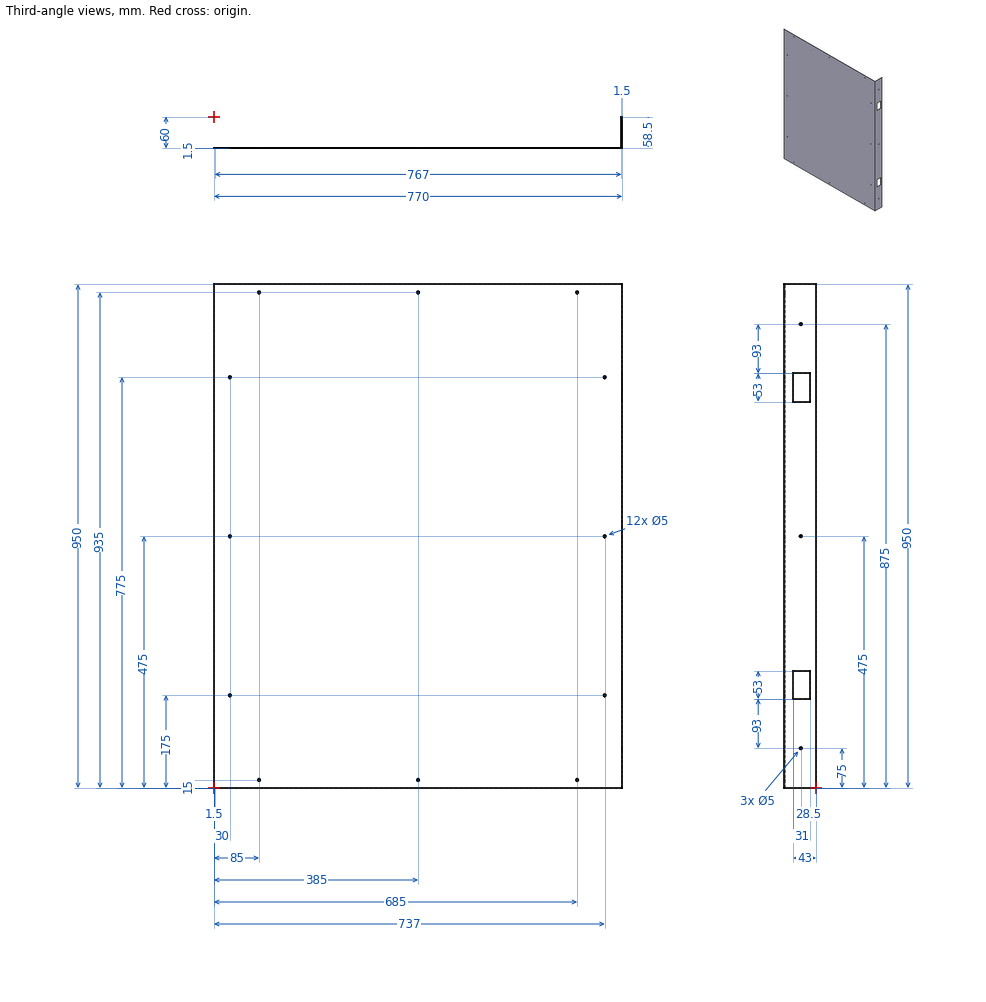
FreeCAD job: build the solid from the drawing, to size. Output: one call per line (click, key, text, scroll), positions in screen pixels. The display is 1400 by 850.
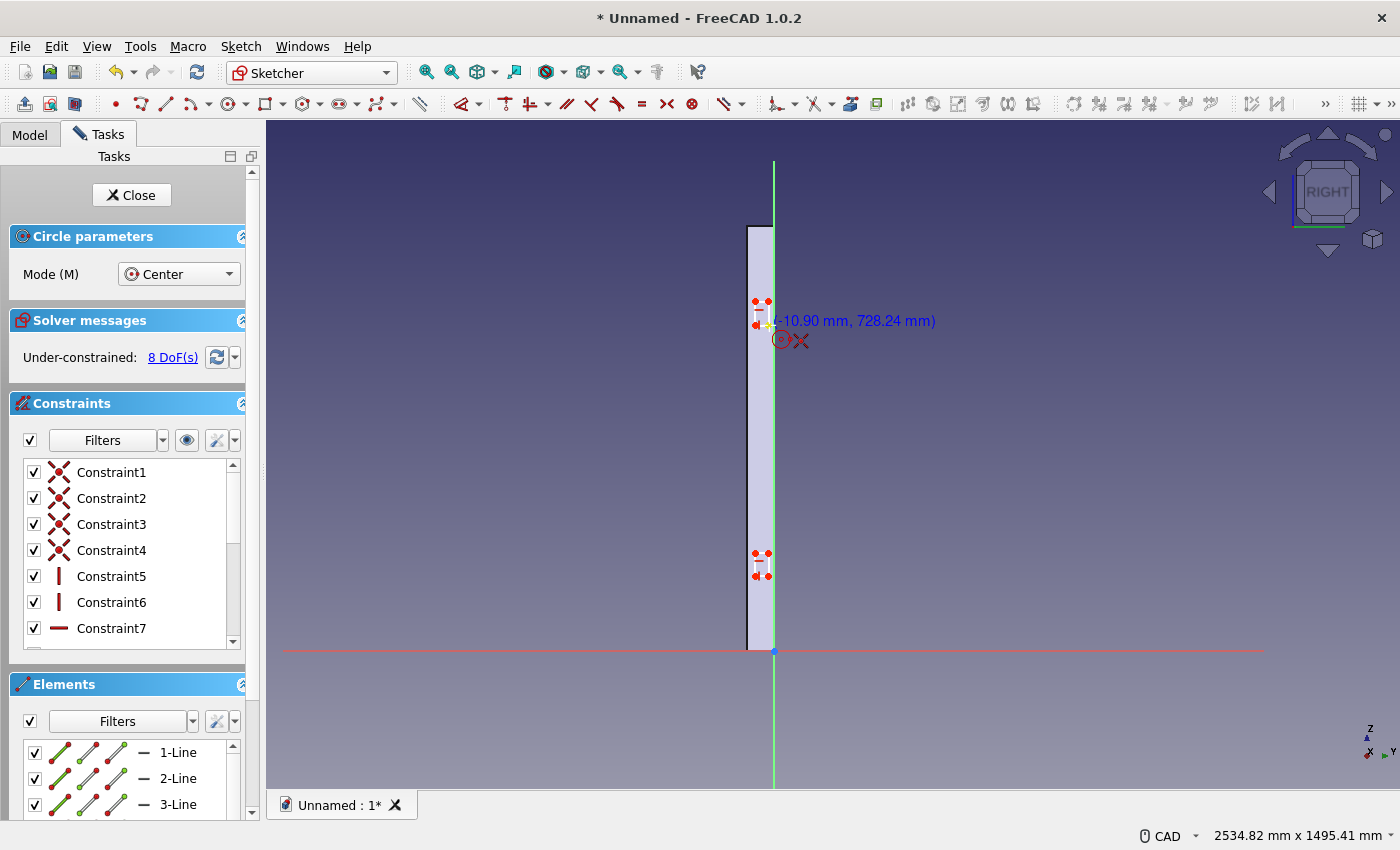
scroll(761, 618, up, 16)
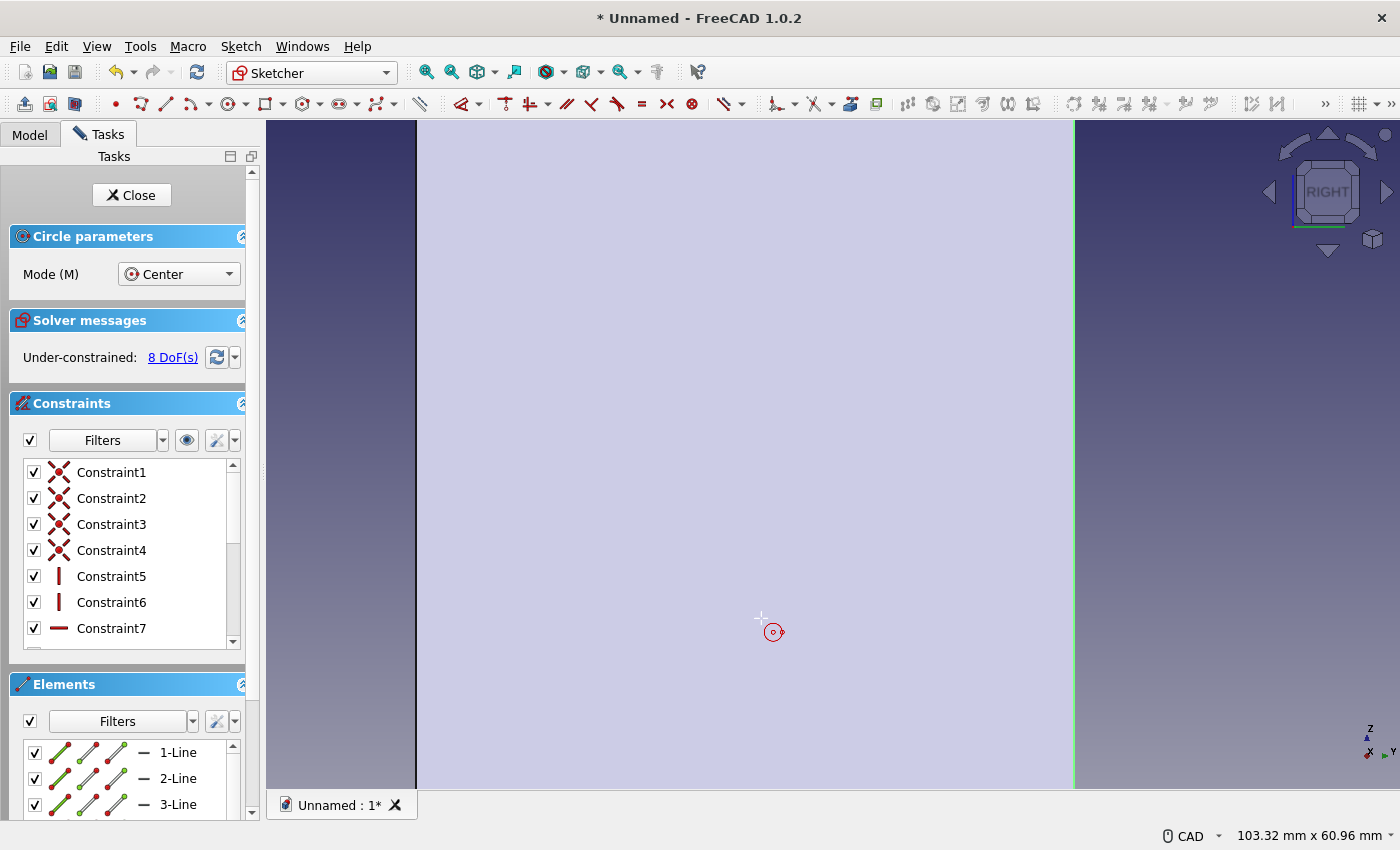
scroll(761, 656, down, 15)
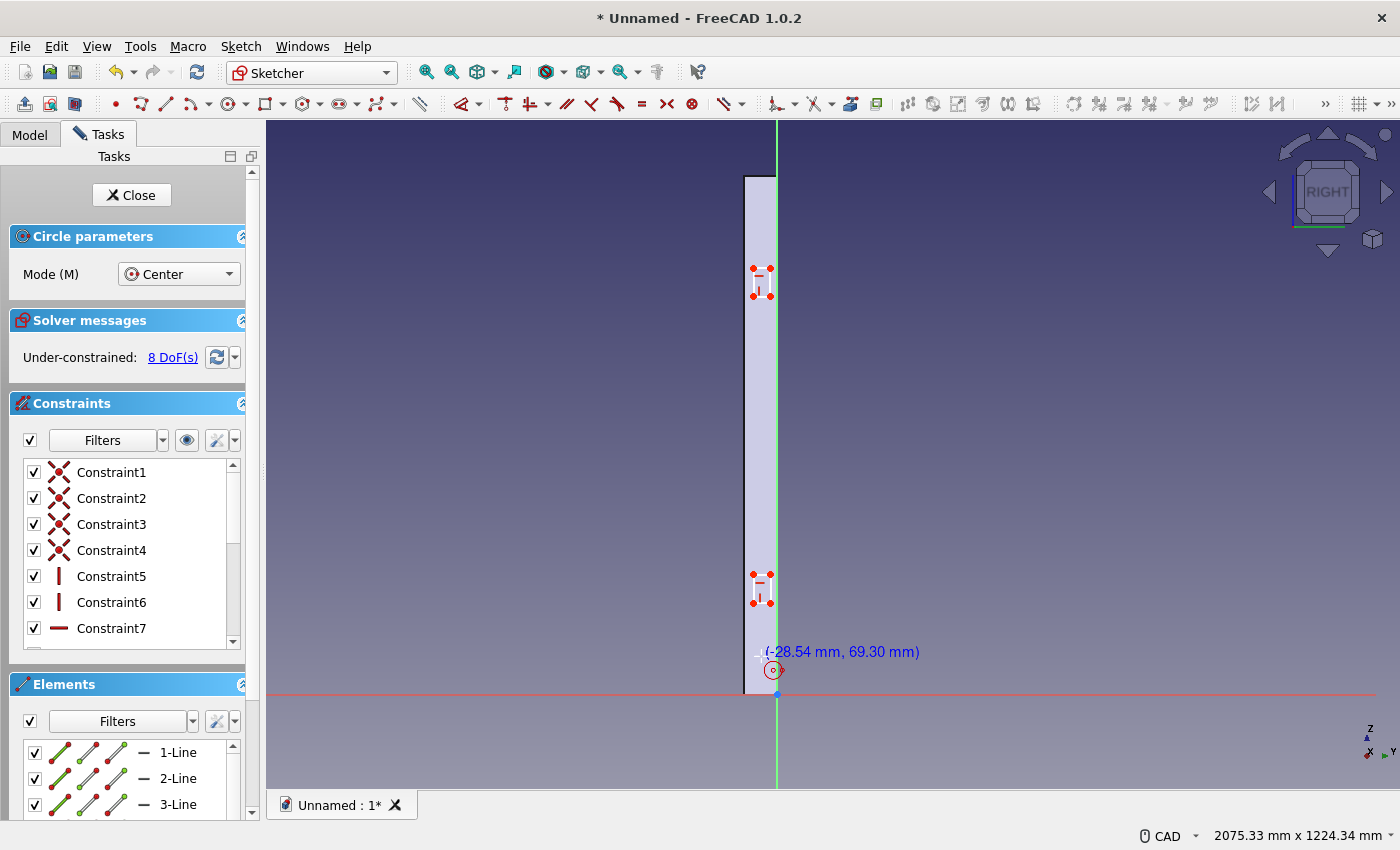
click(761, 654)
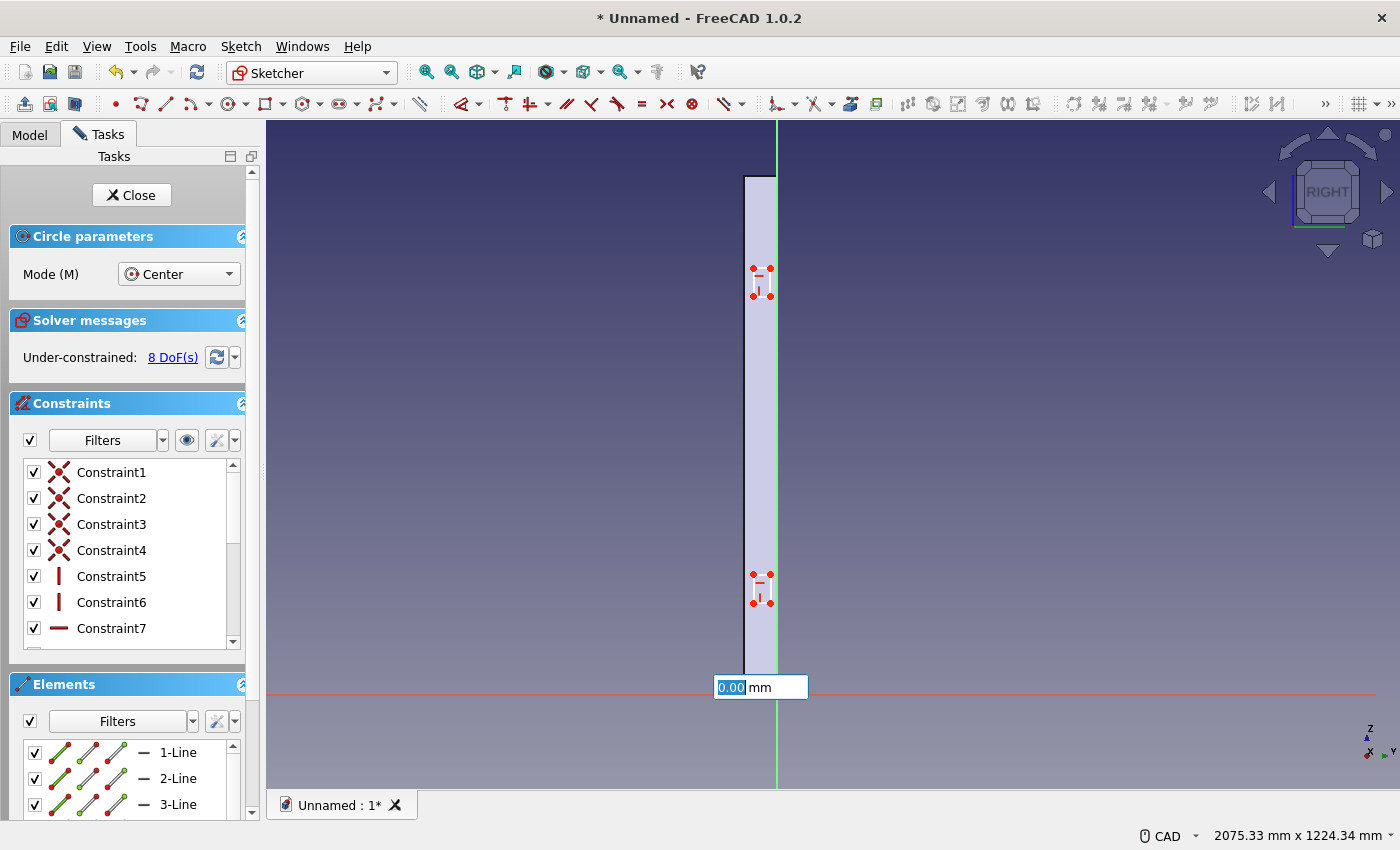
scroll(762, 653, up, 13)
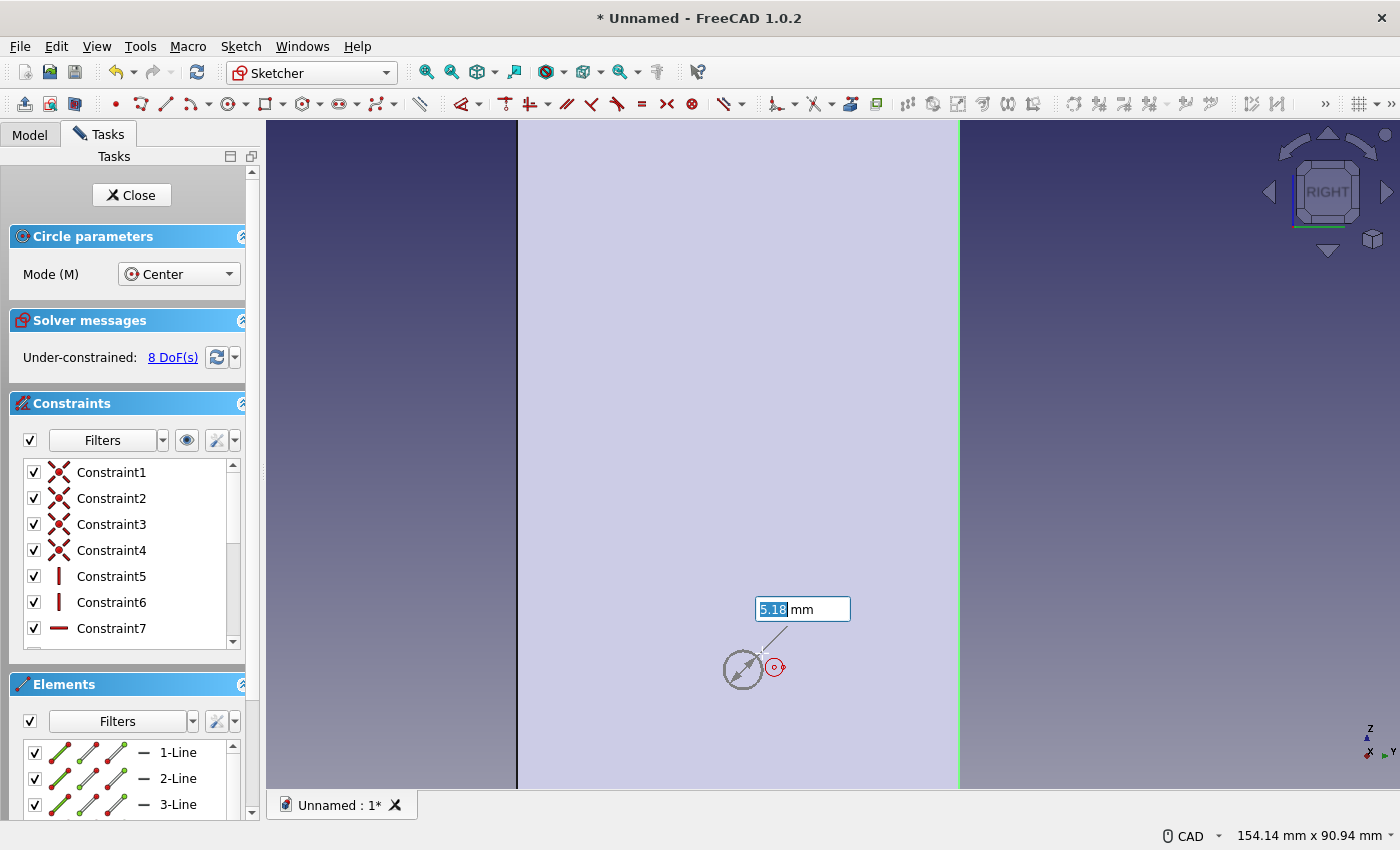
click(762, 639)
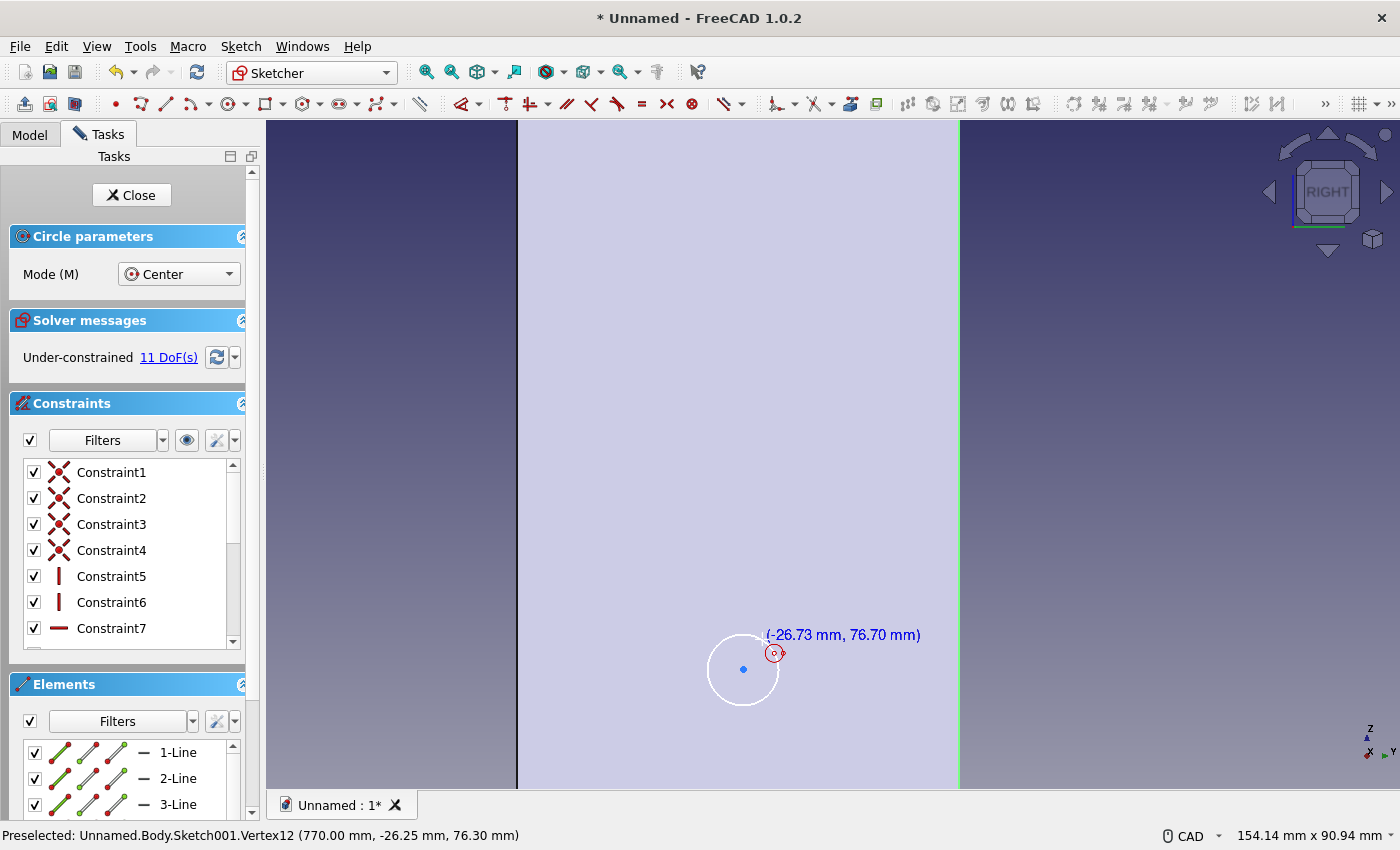
scroll(762, 615, down, 14)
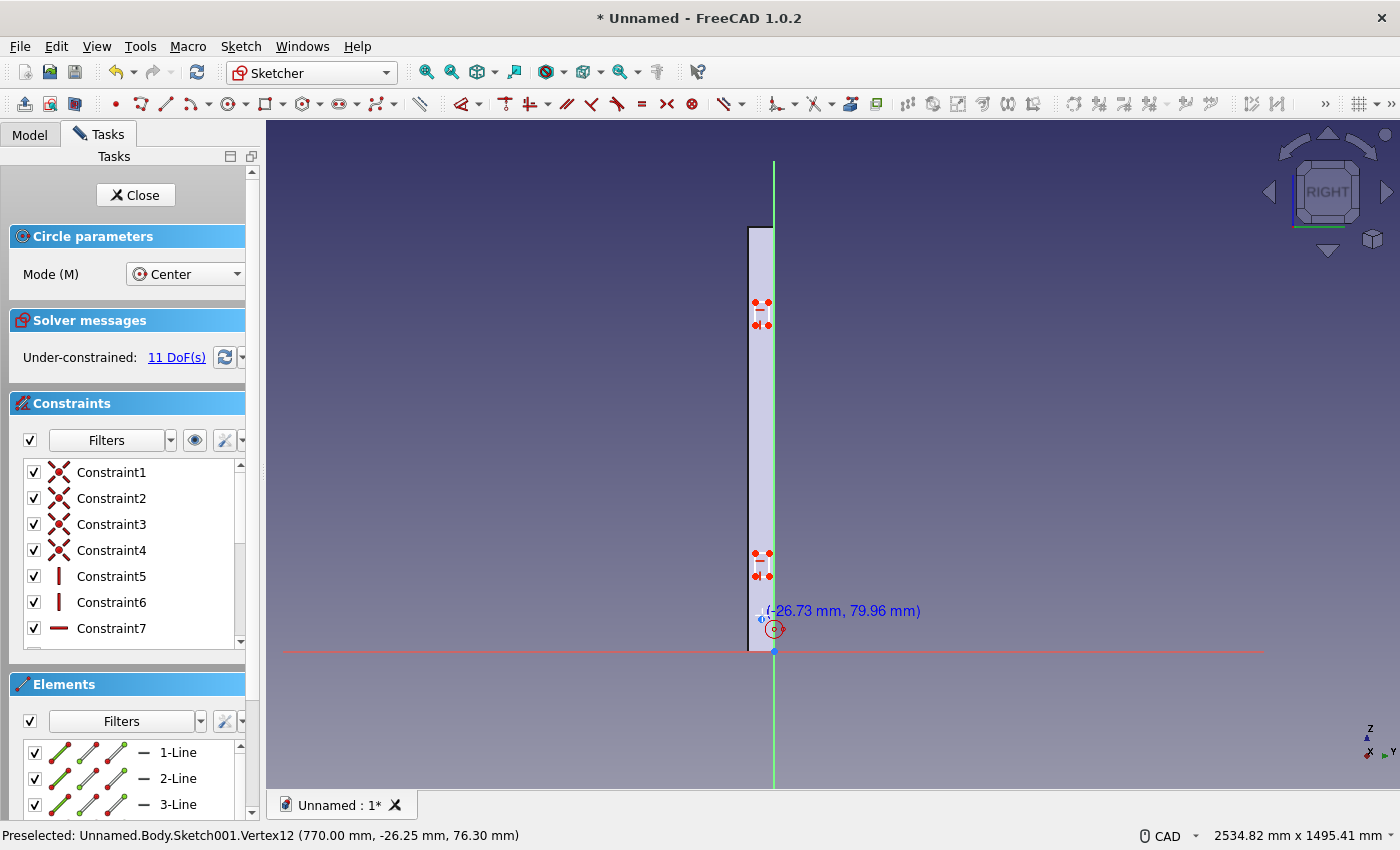
scroll(762, 439, up, 16)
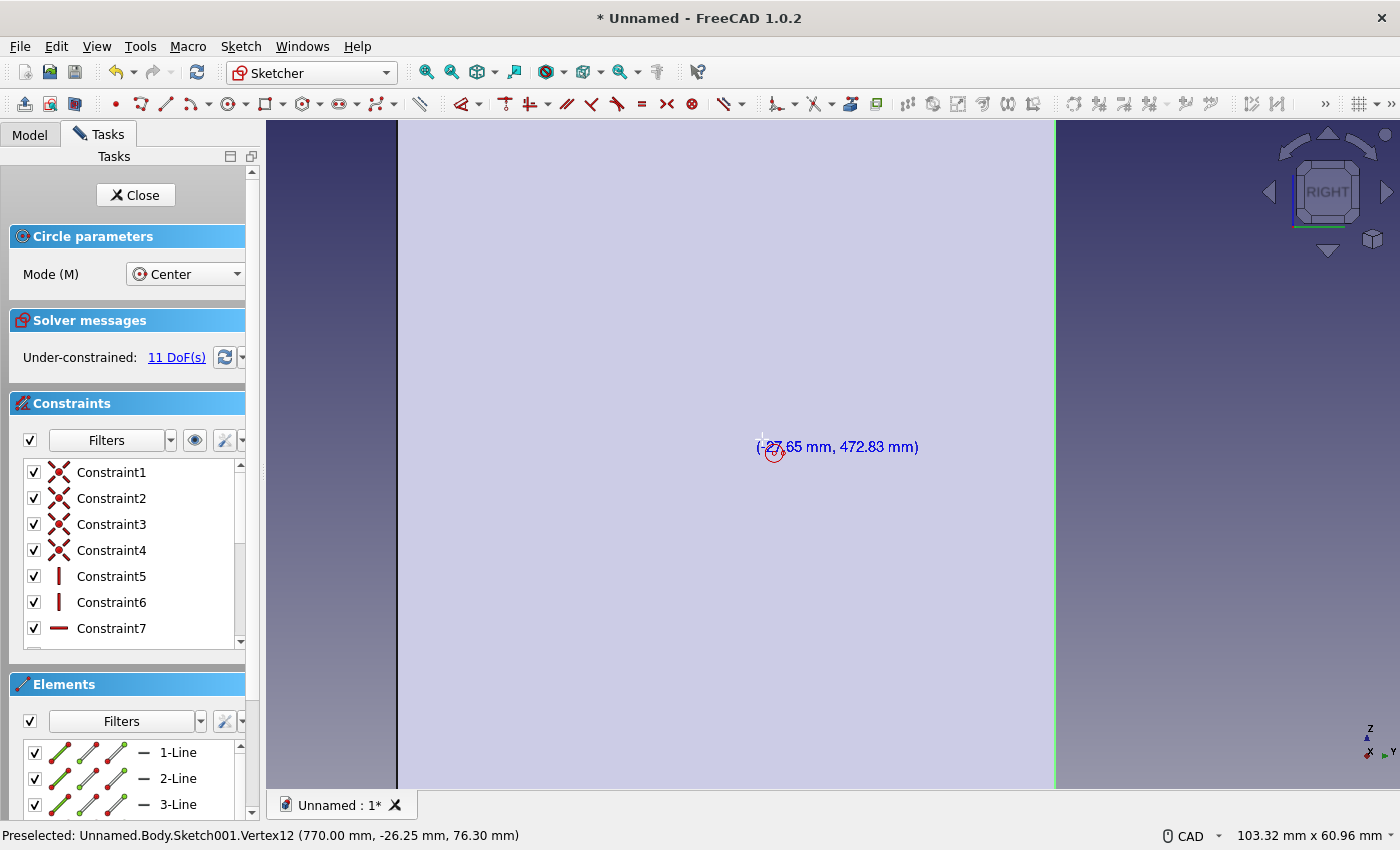
scroll(762, 435, down, 15)